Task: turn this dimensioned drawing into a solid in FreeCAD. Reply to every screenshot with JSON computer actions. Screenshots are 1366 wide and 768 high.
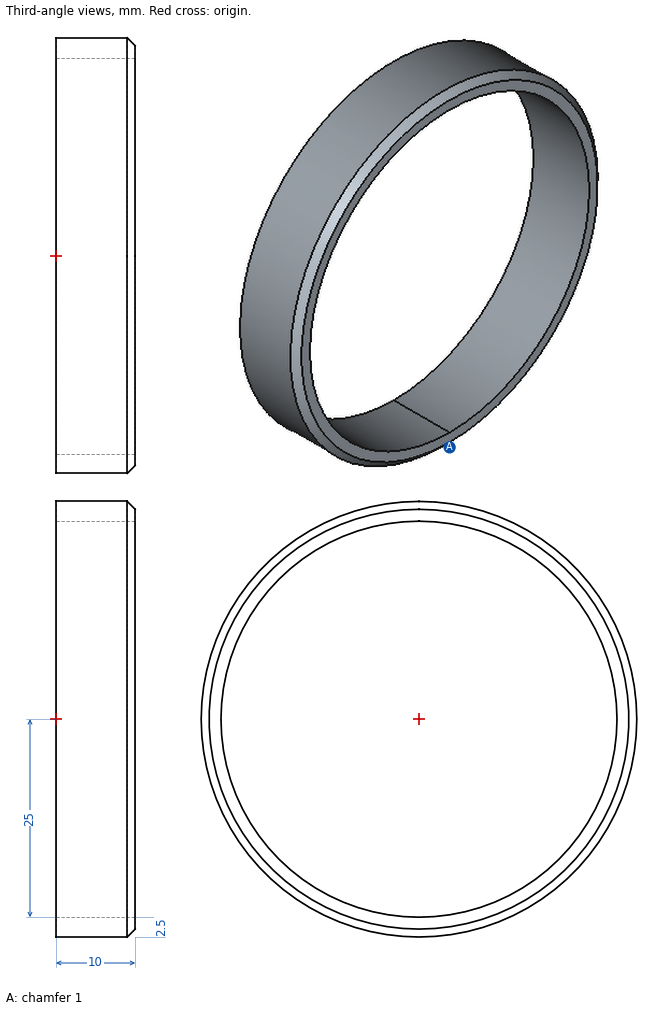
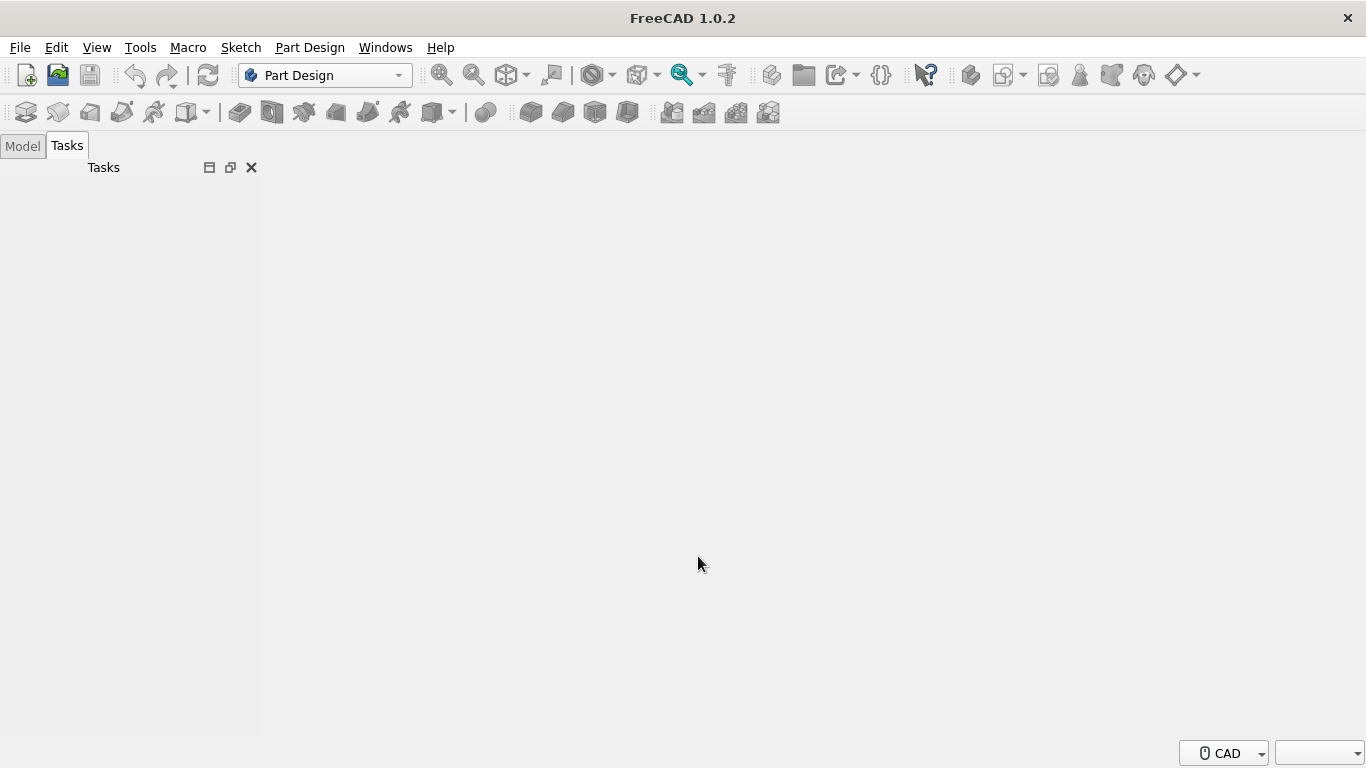
{"action": "left_click", "coordinate": [26, 76]}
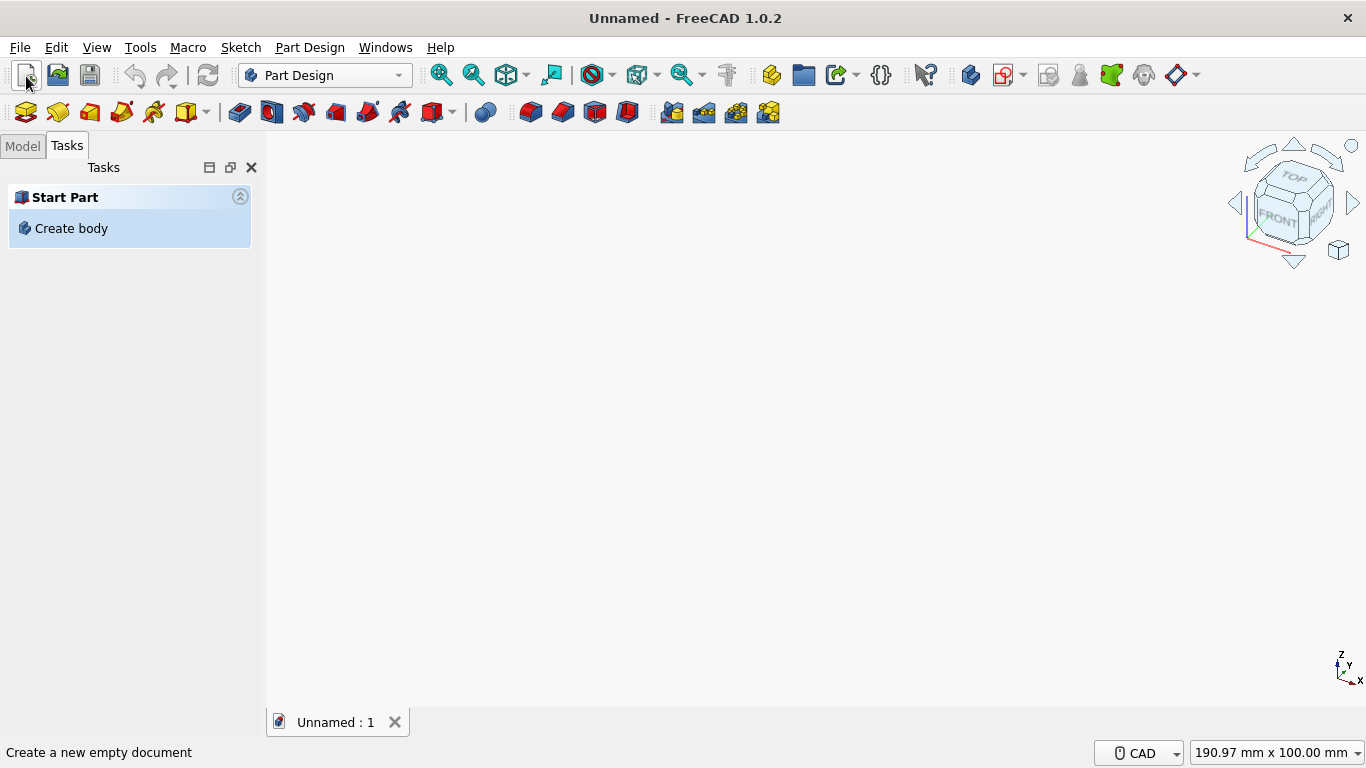
{"action": "left_click", "coordinate": [1004, 76]}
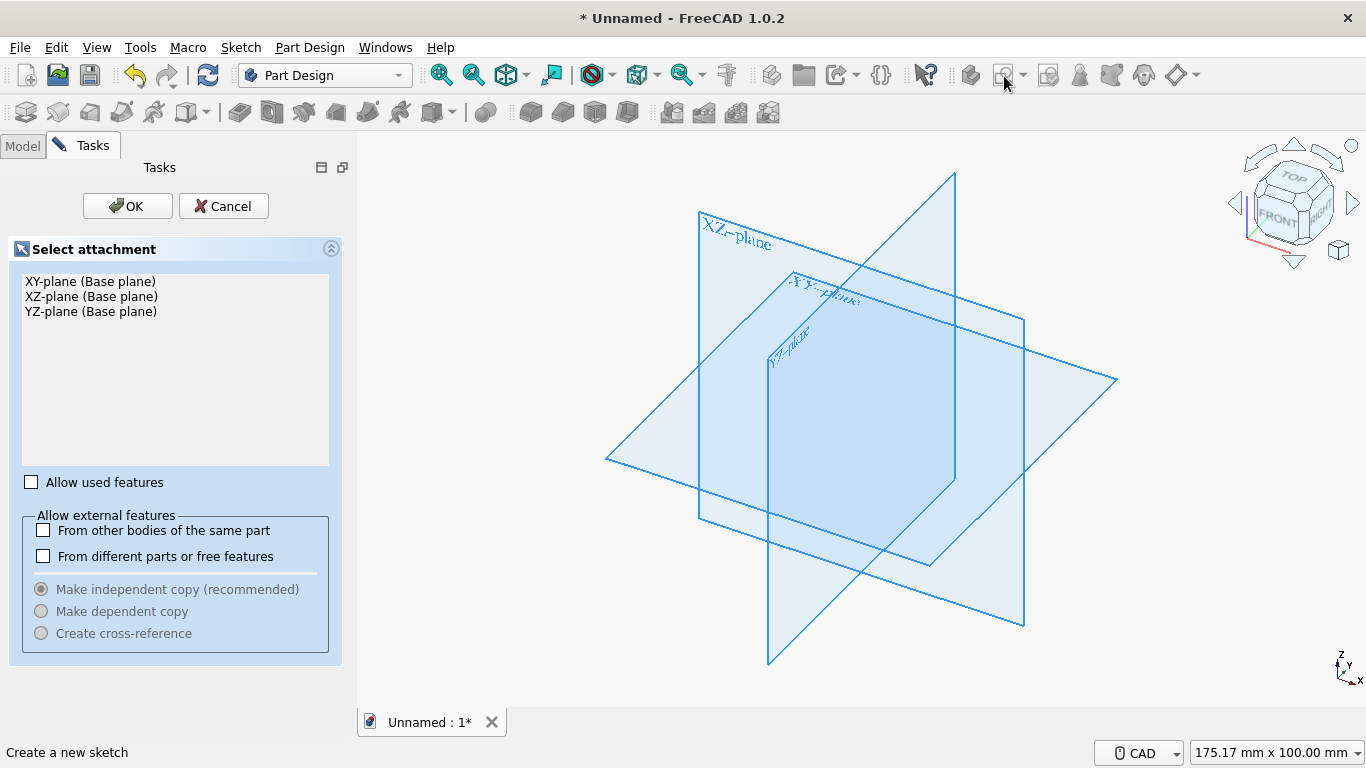
{"action": "left_click", "coordinate": [82, 296]}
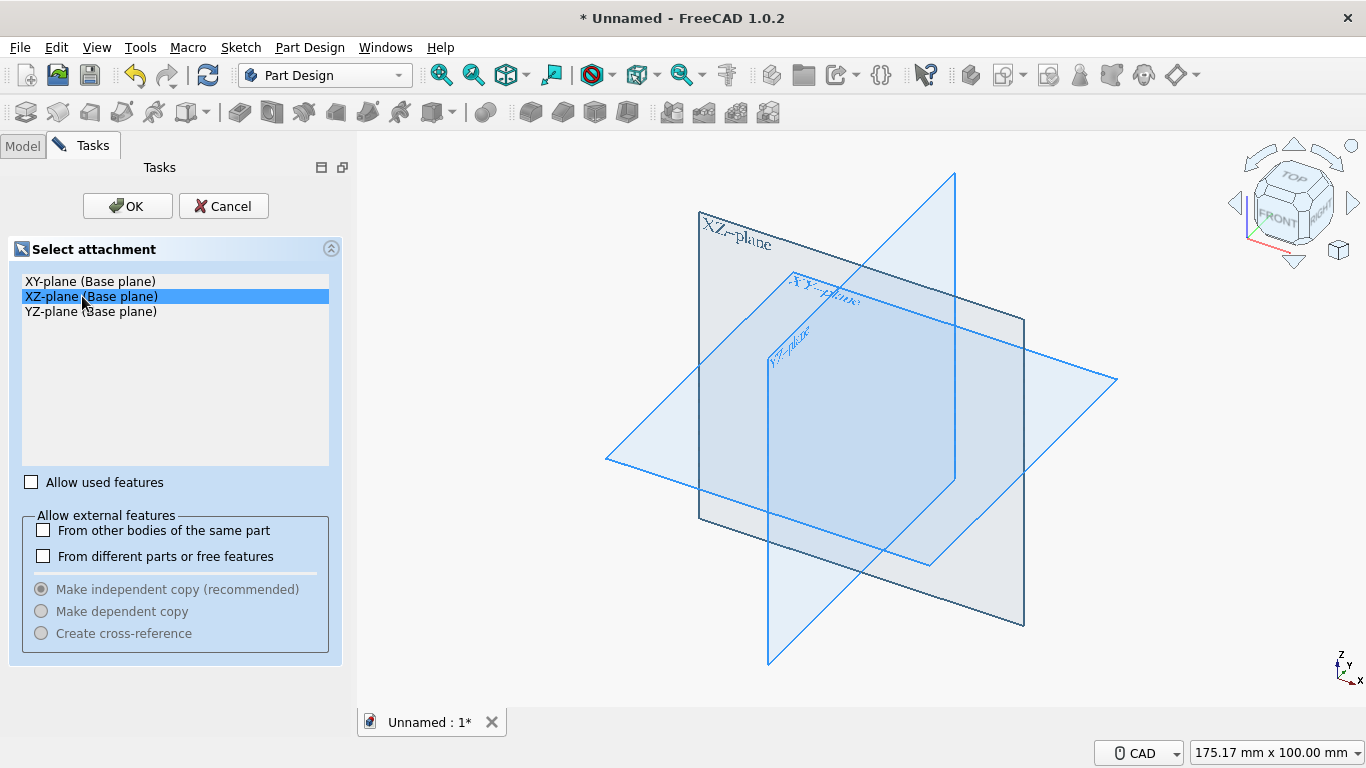
{"action": "left_click", "coordinate": [128, 206]}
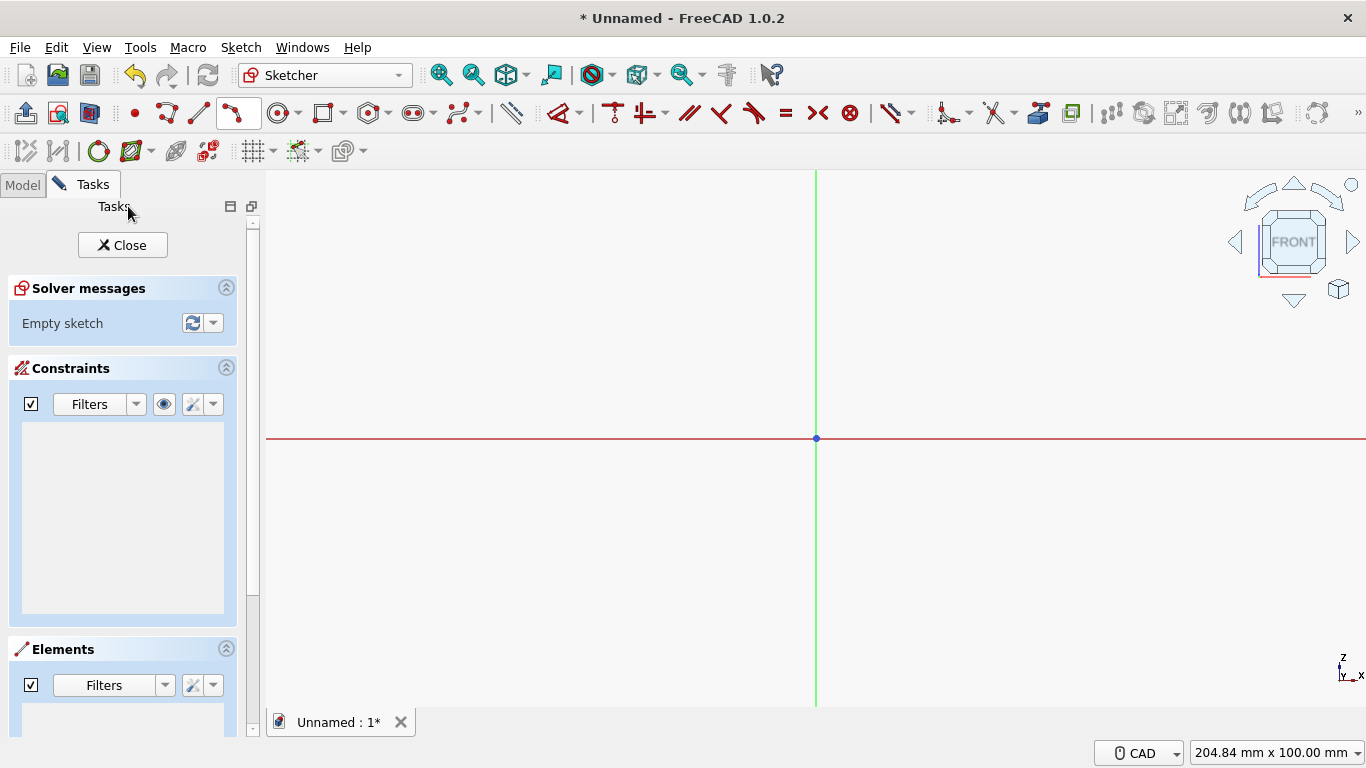
{"action": "scroll", "coordinate": [852, 594], "scroll_direction": "up", "scroll_amount": 12}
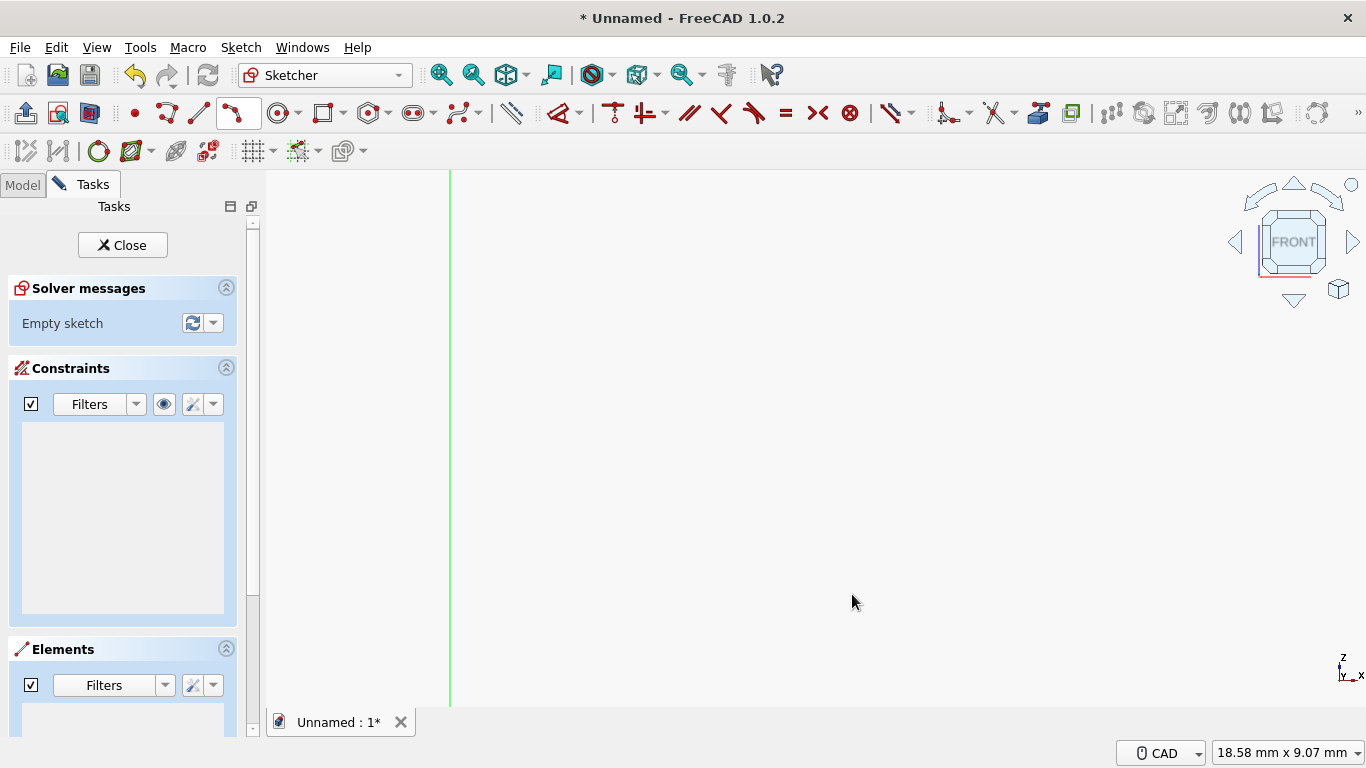
{"action": "key", "text": "g r"}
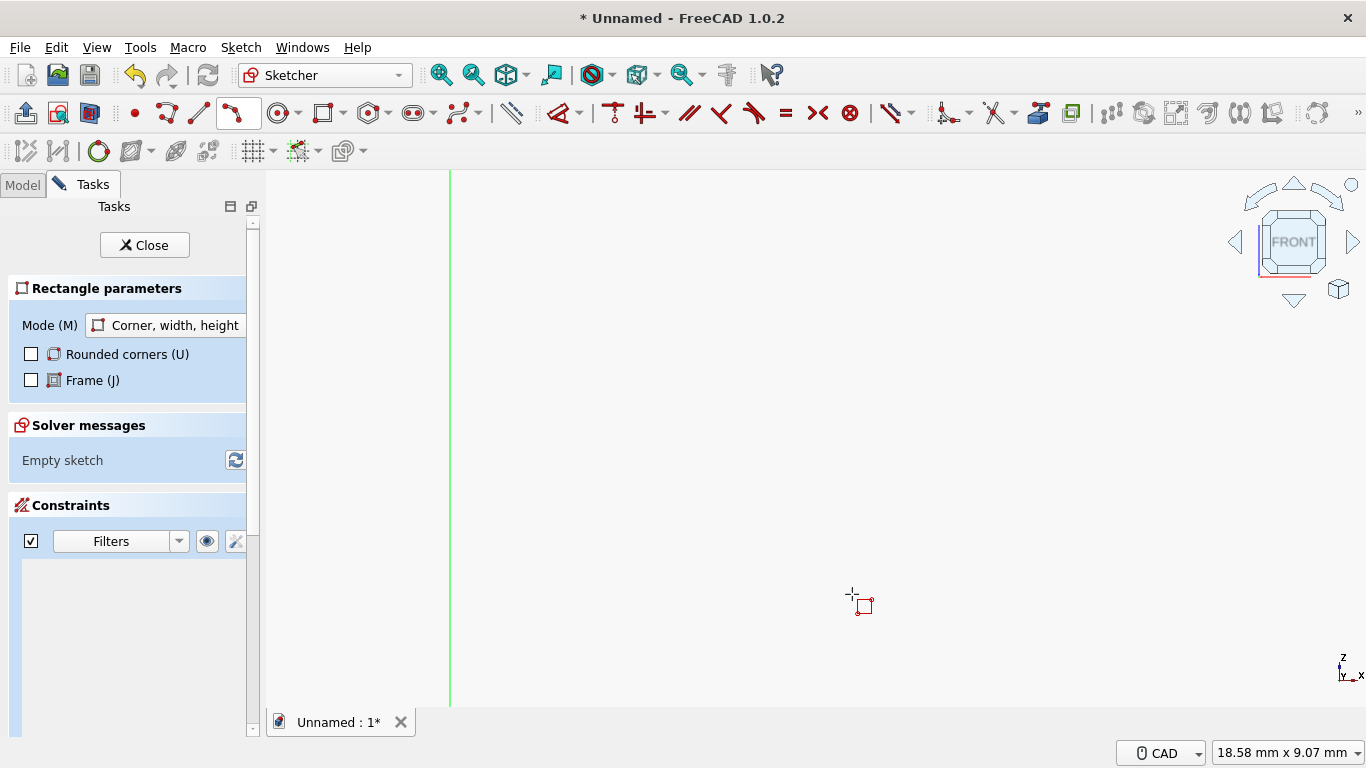
{"action": "left_click", "coordinate": [450, 352]}
{"action": "mouse_move", "coordinate": [1042, 500]}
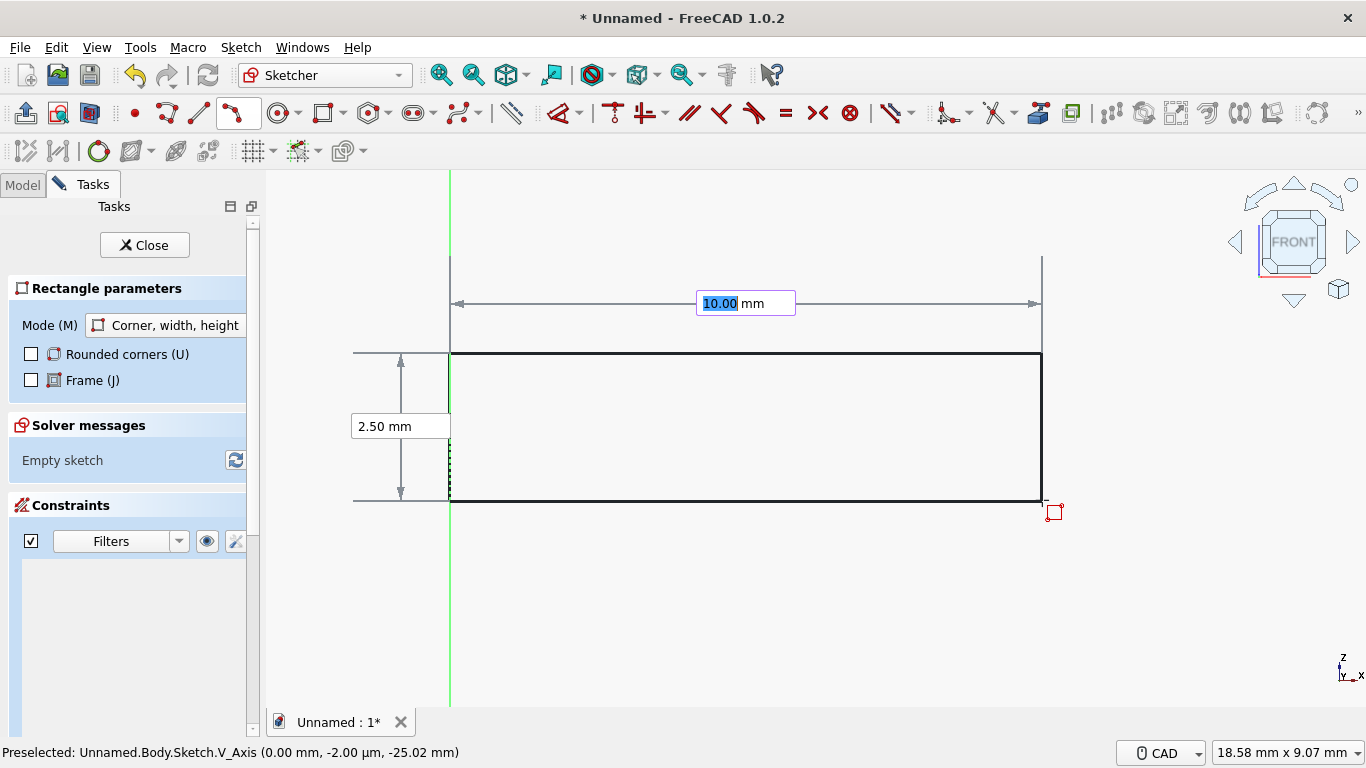
{"action": "type", "text": "10"}
{"action": "key", "text": "Tab"}
{"action": "type", "text": "2.5"}
{"action": "key", "text": "Return"}
{"action": "key", "text": "Escape"}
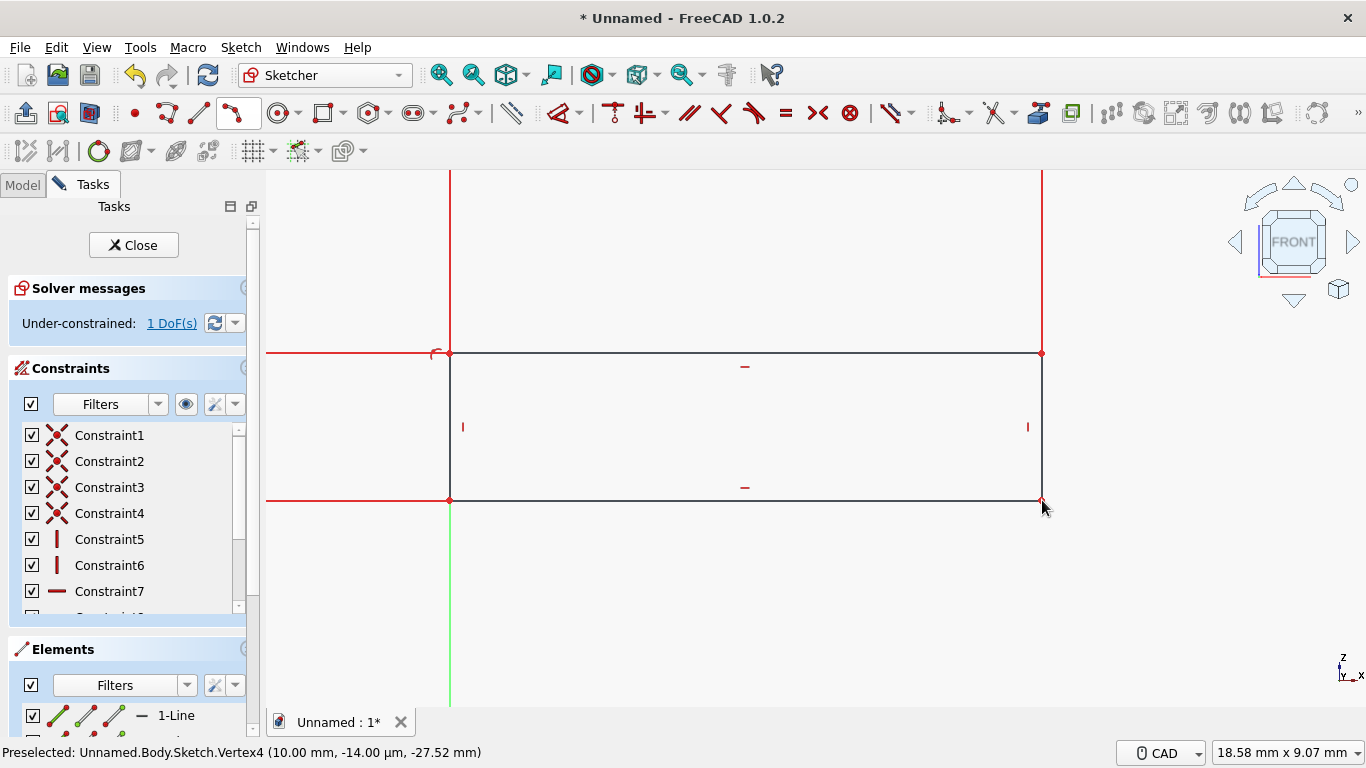
{"action": "left_click", "coordinate": [558, 114]}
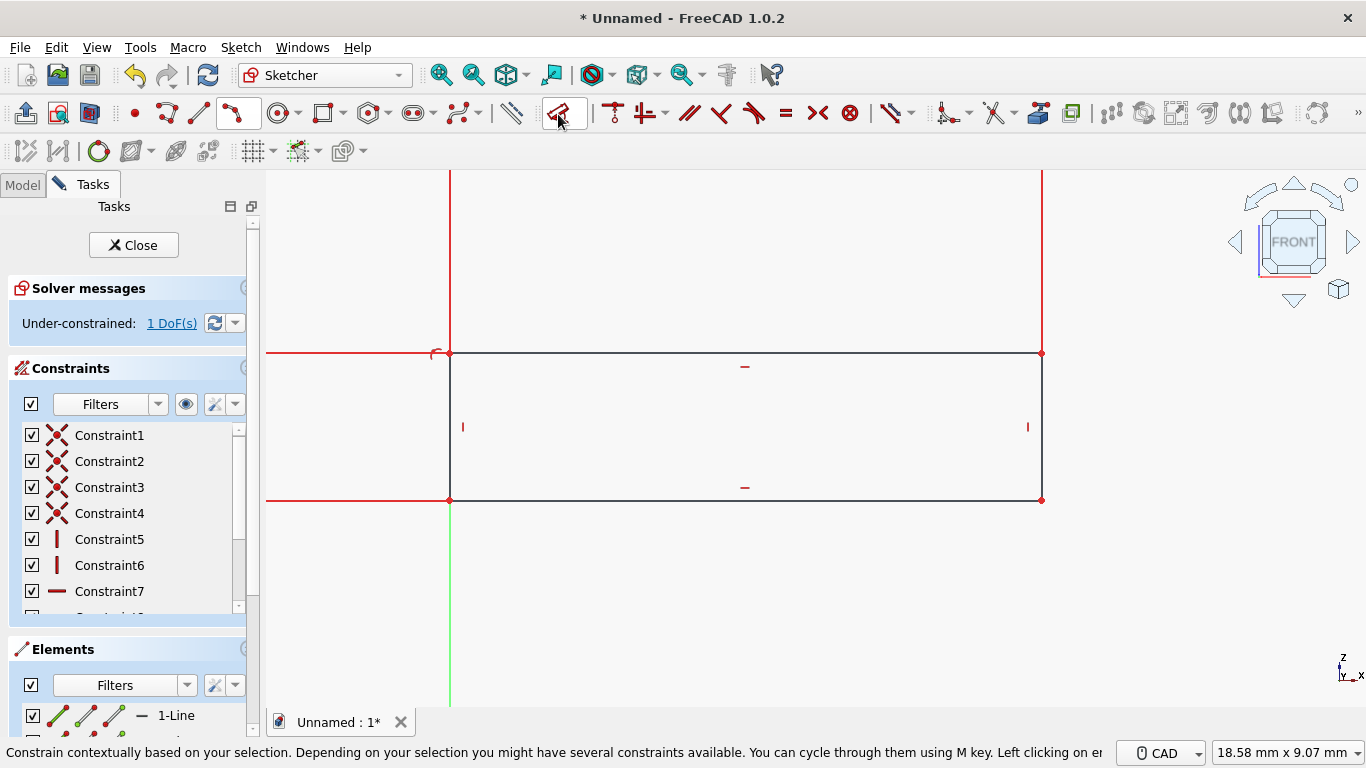
{"action": "left_click", "coordinate": [450, 353]}
{"action": "left_click", "coordinate": [416, 275]}